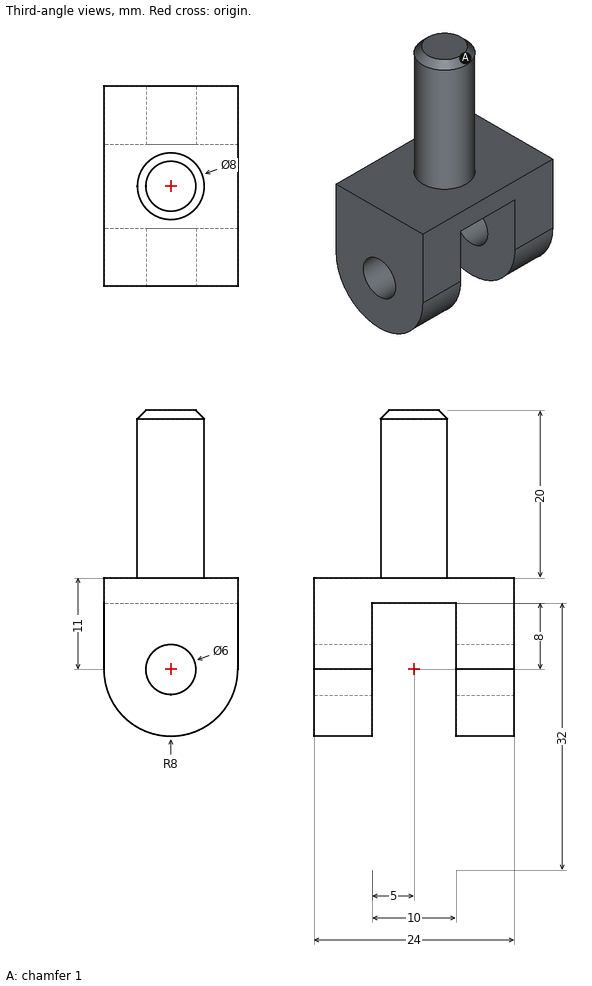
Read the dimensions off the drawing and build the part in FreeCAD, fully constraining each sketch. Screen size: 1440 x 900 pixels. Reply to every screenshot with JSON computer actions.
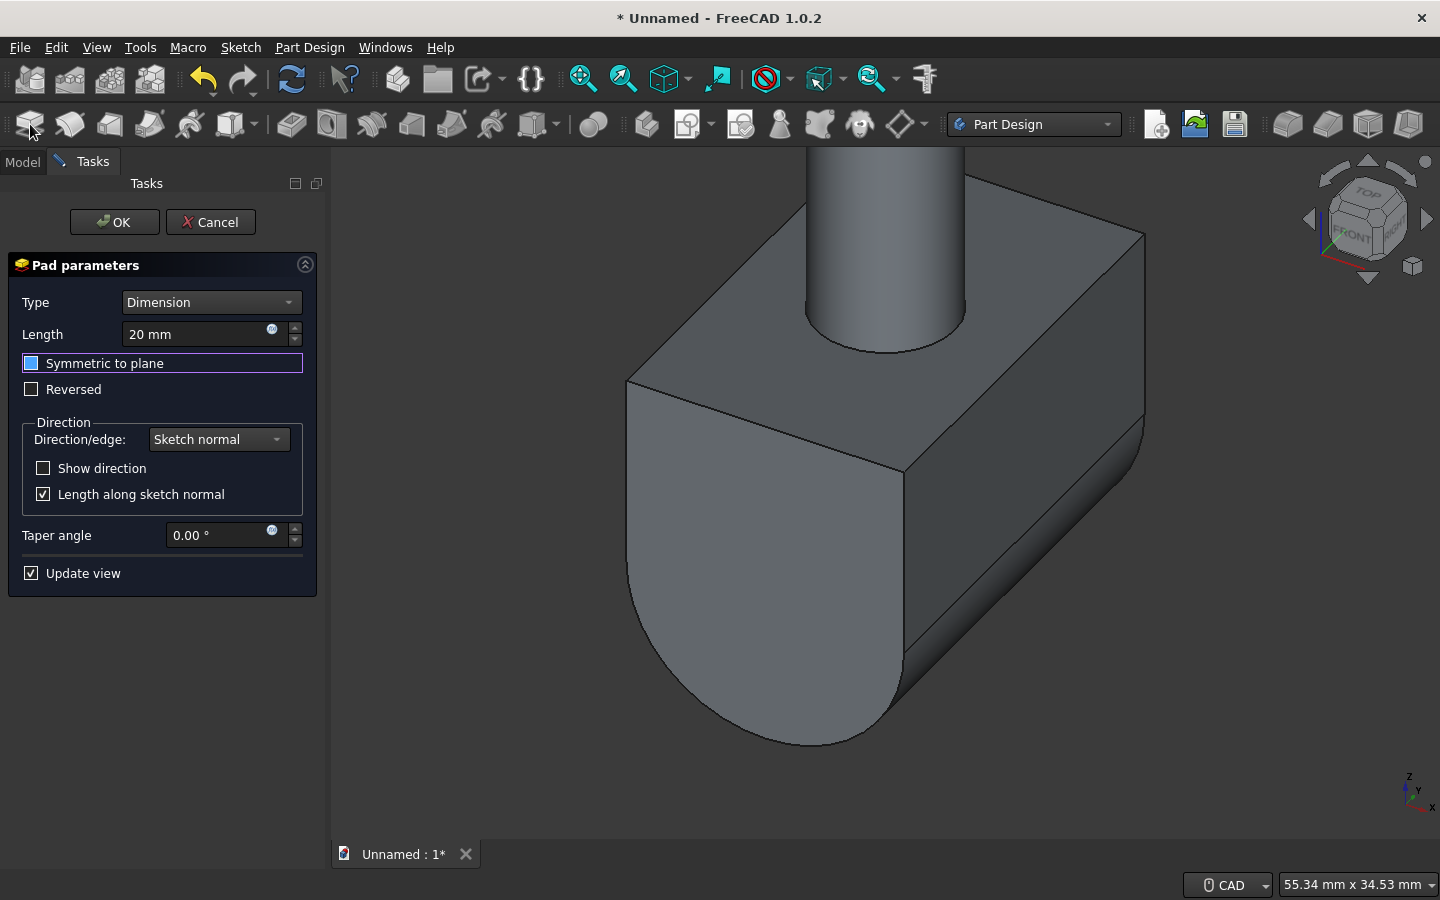
{"action": "left_click", "coordinate": [115, 222]}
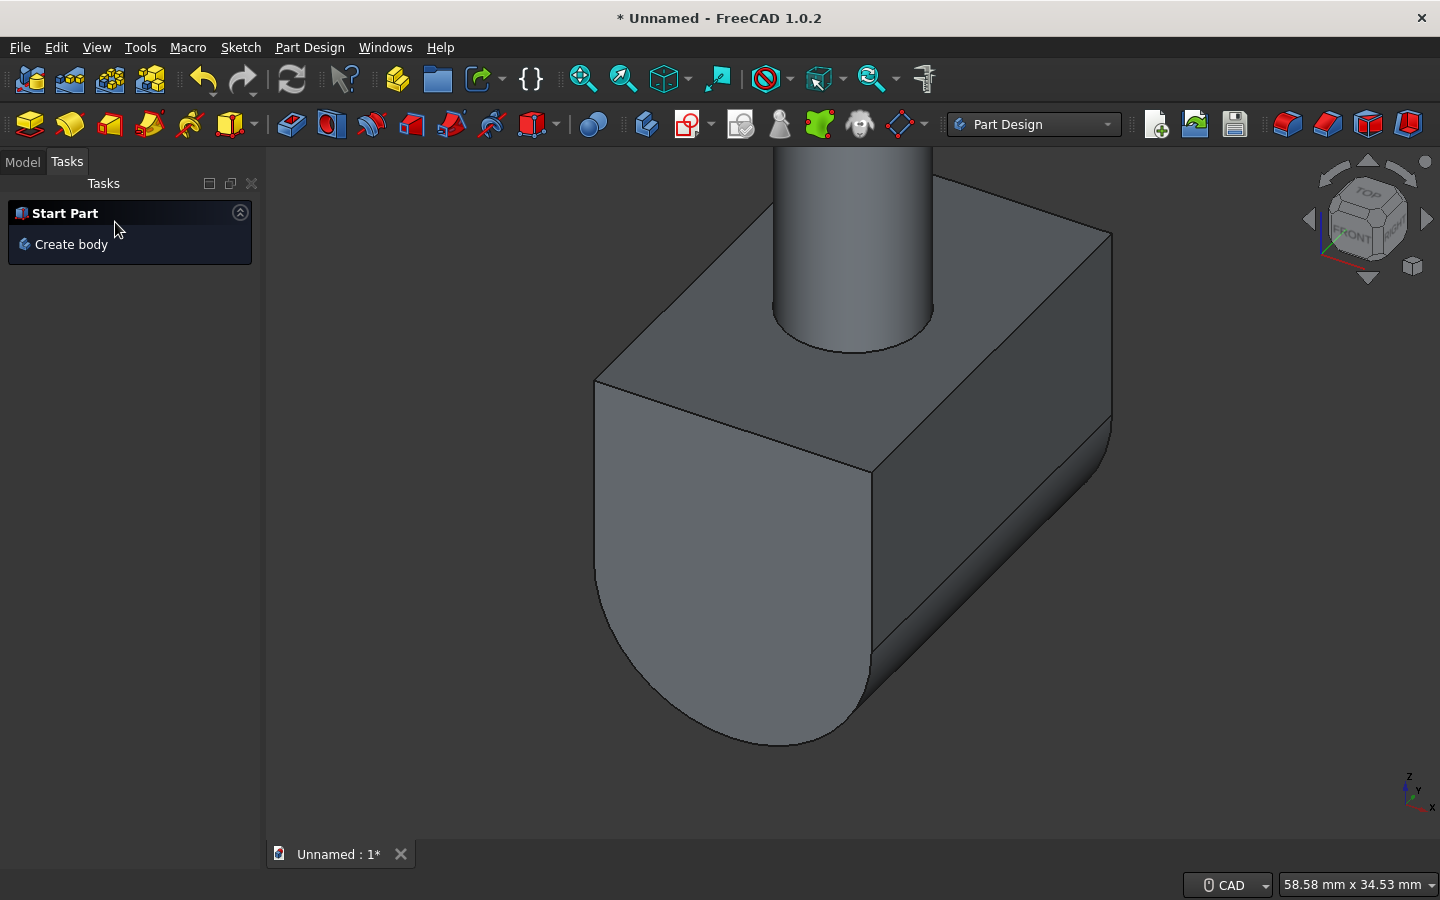
{"action": "left_click", "coordinate": [584, 80]}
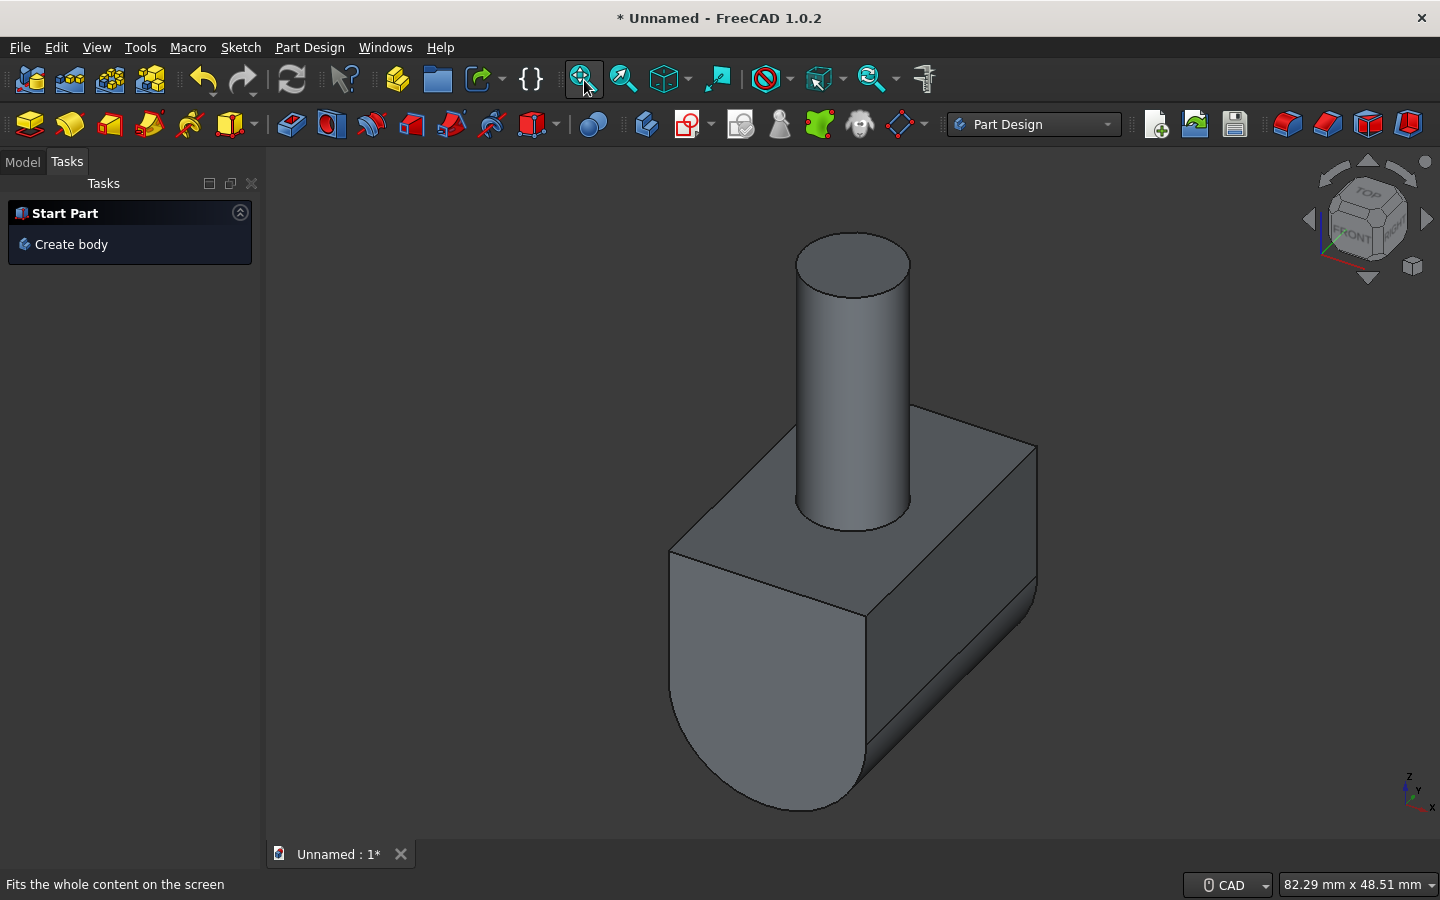
{"action": "left_click", "coordinate": [952, 595]}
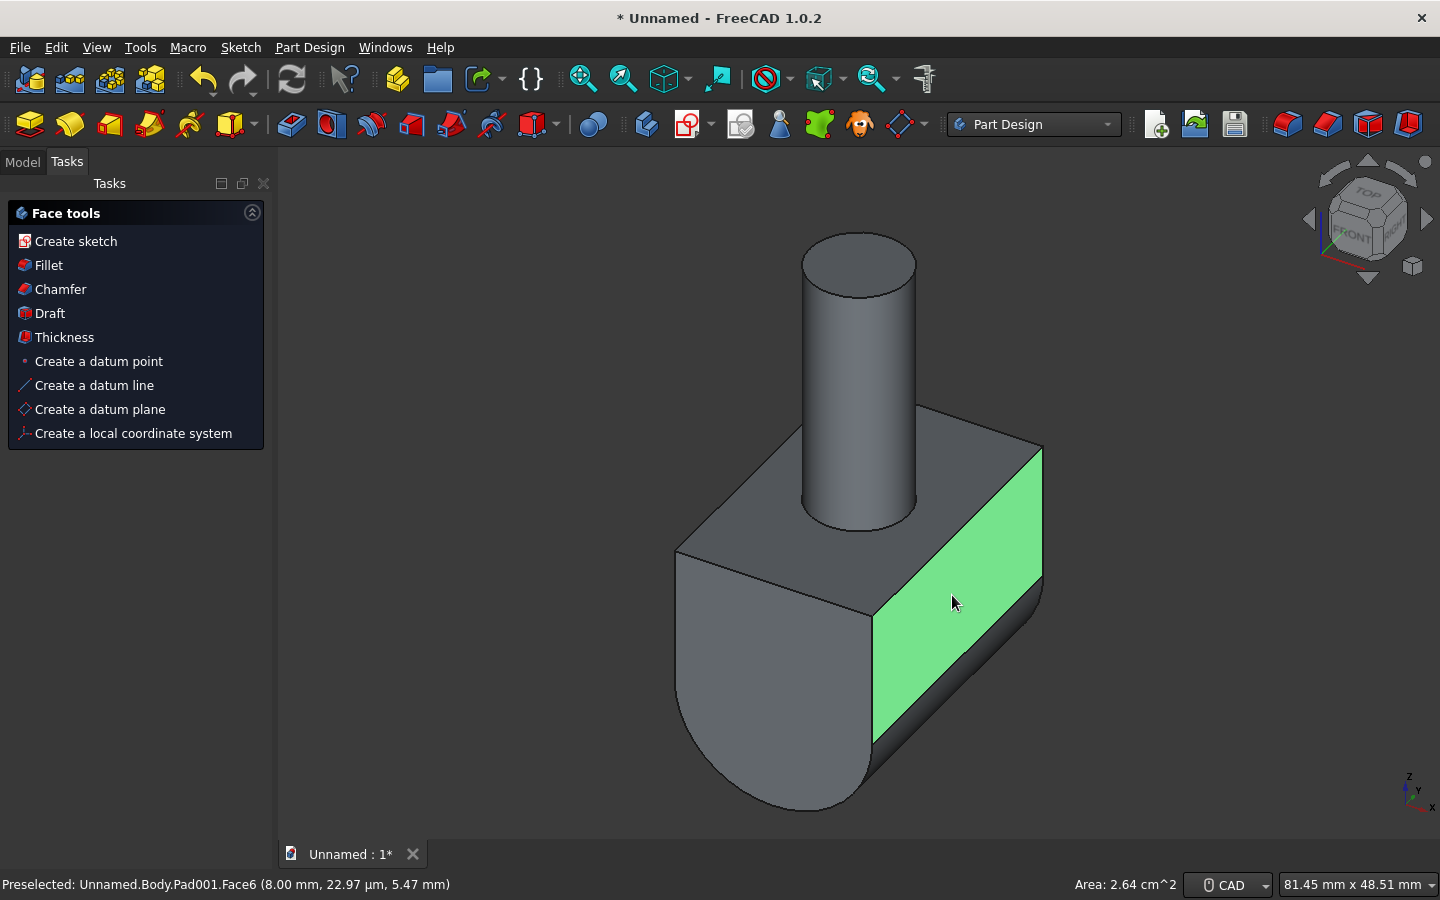
{"action": "left_click", "coordinate": [688, 124]}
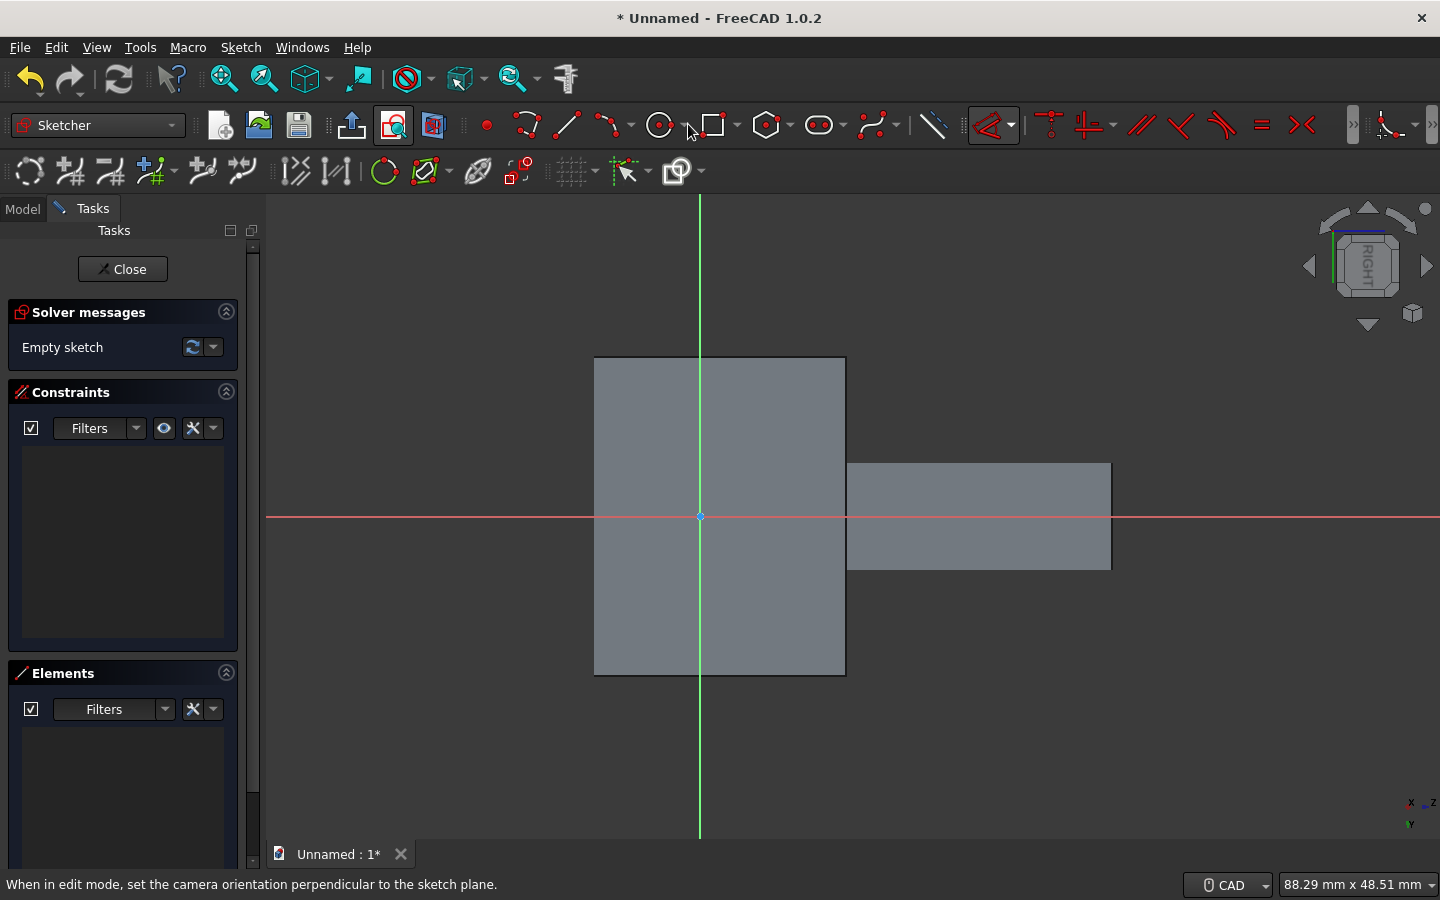
{"action": "scroll", "coordinate": [294, 517], "scroll_direction": "up", "scroll_amount": 2}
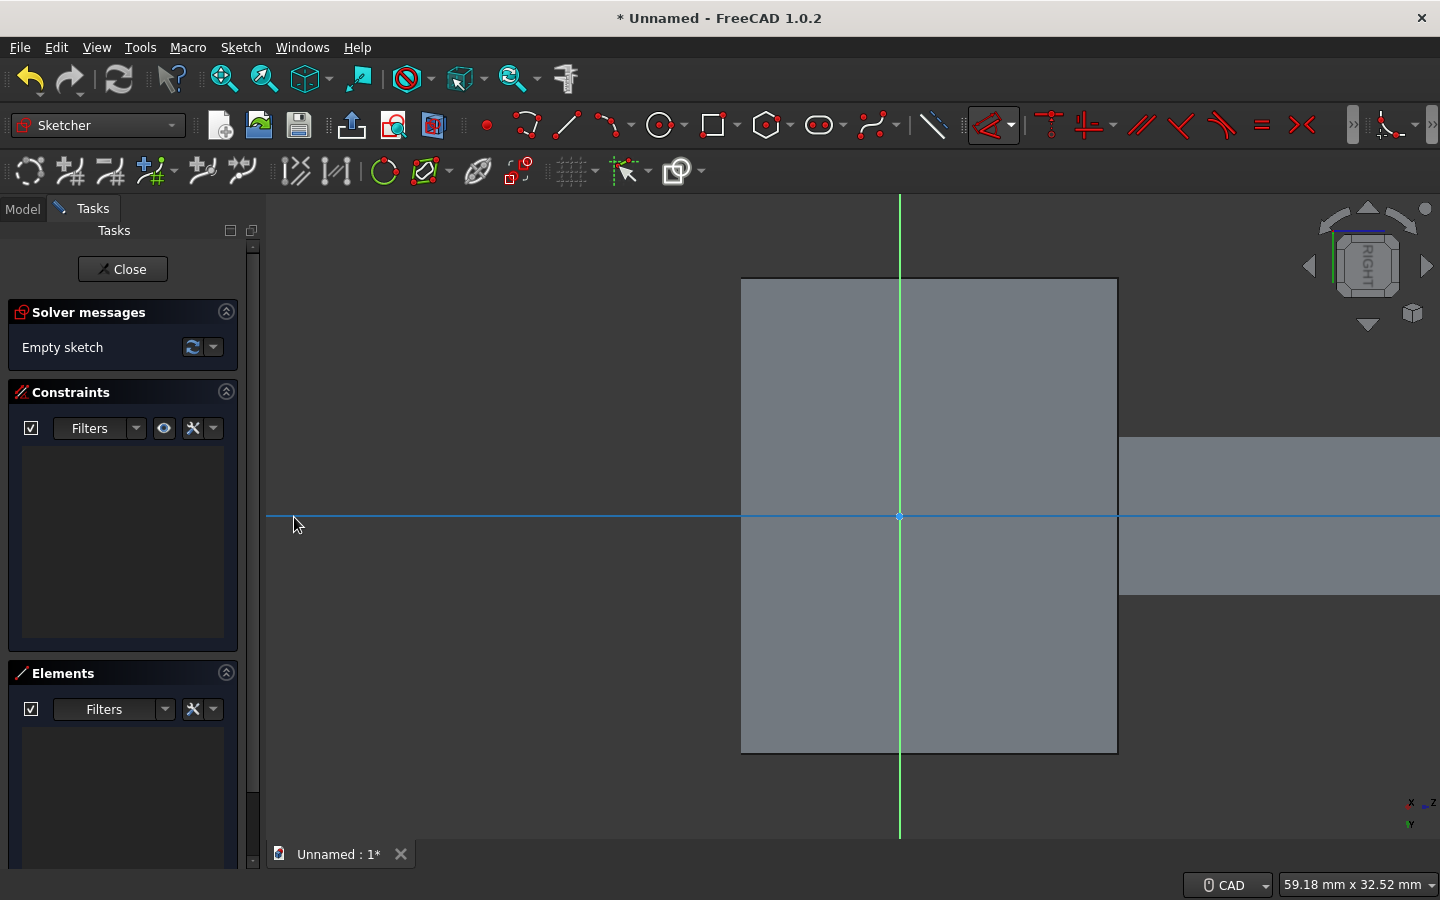
{"action": "left_click", "coordinate": [714, 126]}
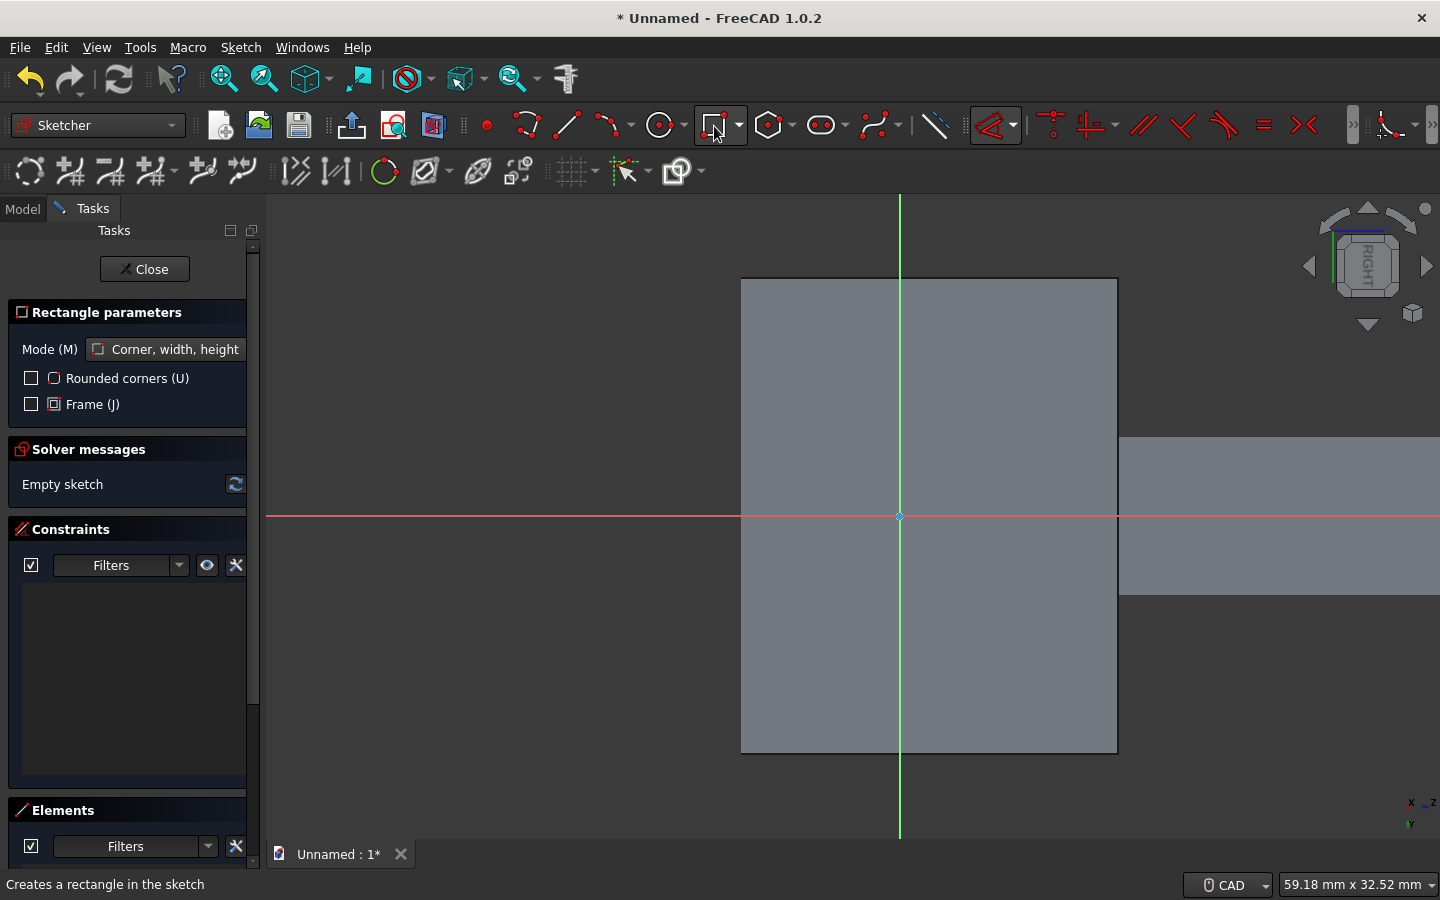
{"action": "left_click", "coordinate": [424, 417]}
{"action": "left_click", "coordinate": [1058, 615]}
{"action": "key", "text": "Escape"}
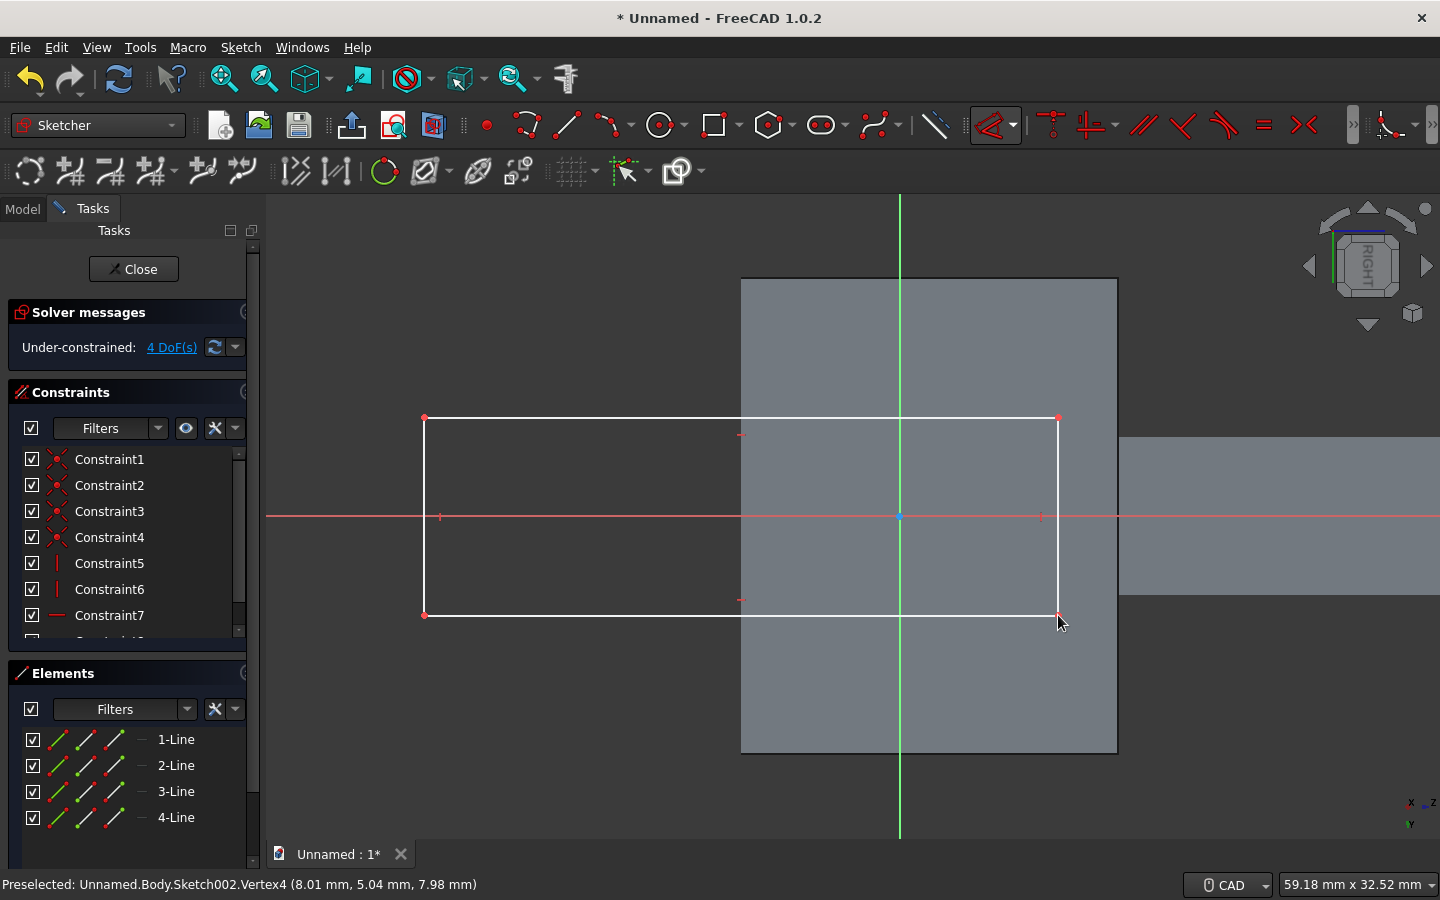
{"action": "left_click", "coordinate": [424, 477]}